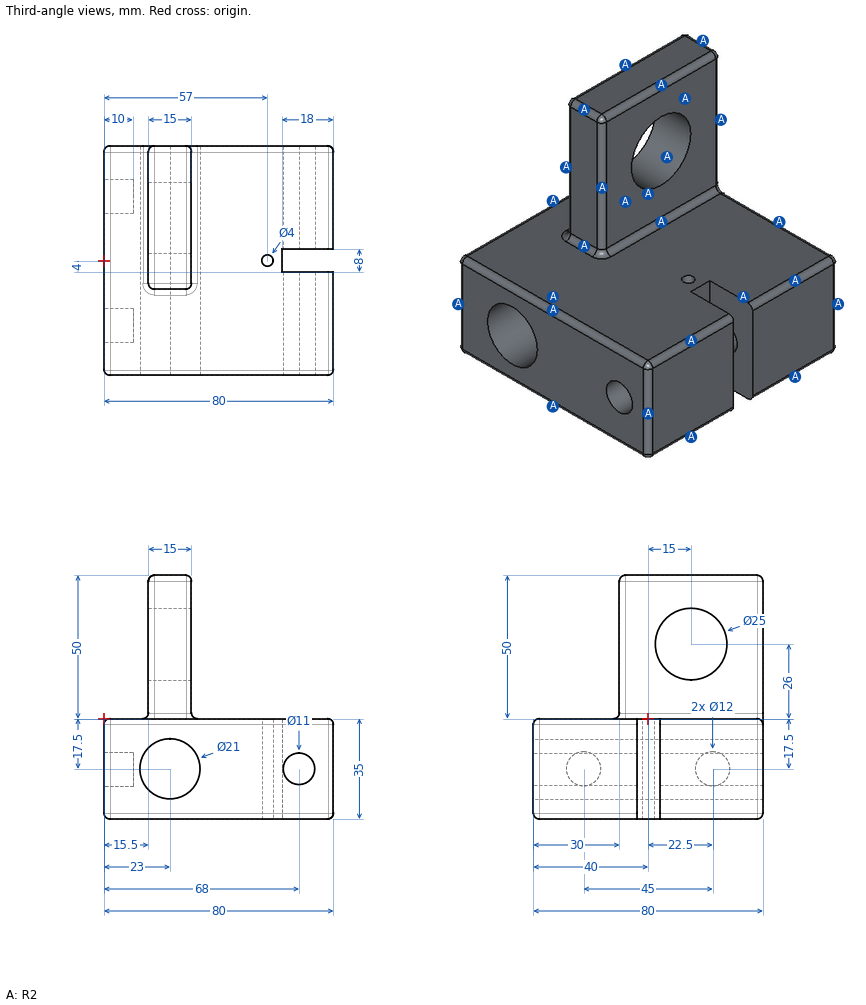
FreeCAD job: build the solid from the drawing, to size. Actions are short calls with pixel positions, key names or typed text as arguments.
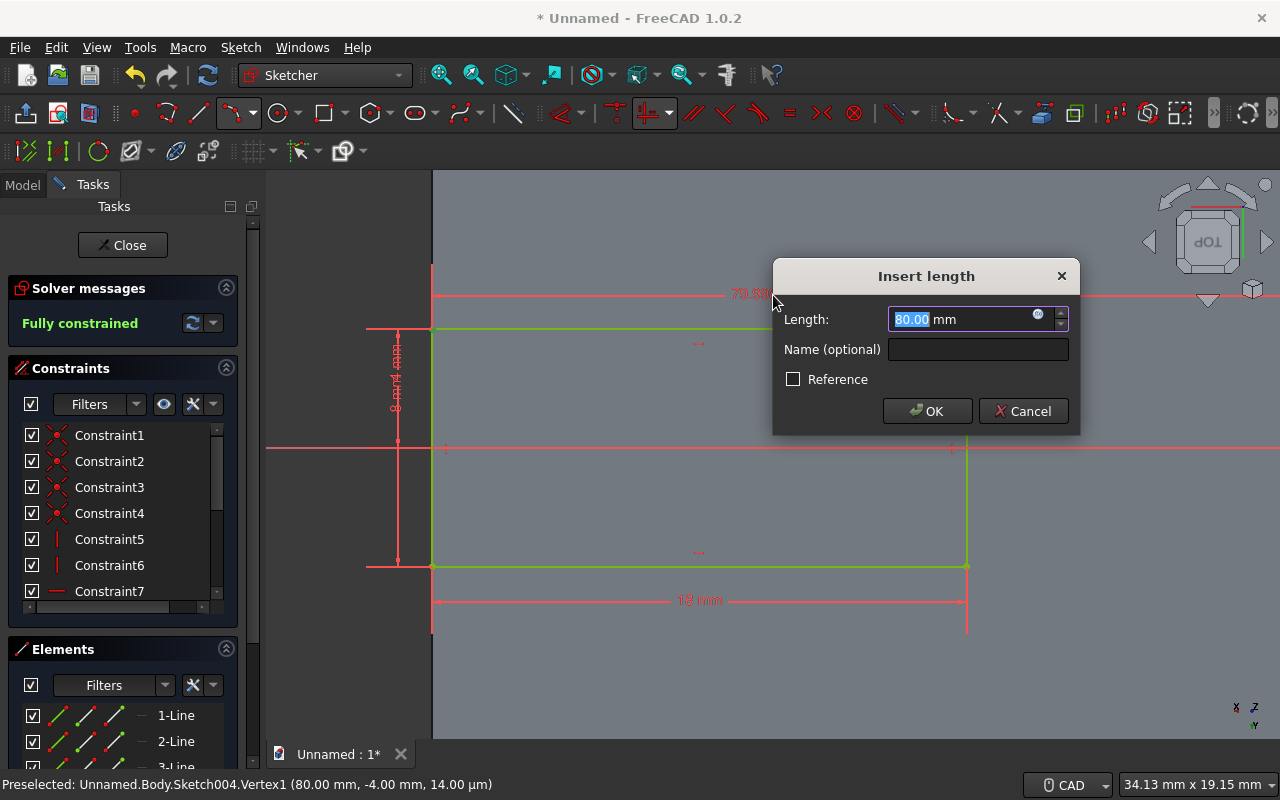
text(80)
key(Return)
key(Escape)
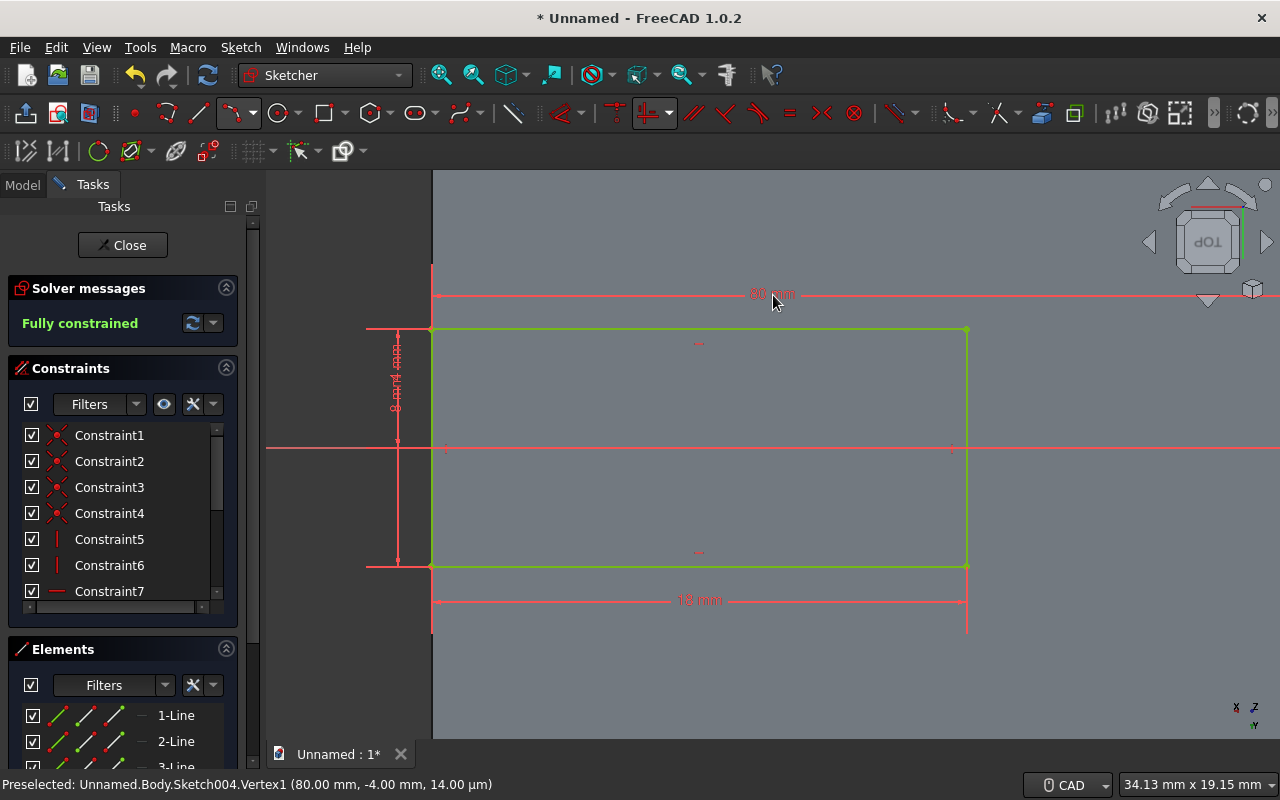
click(123, 245)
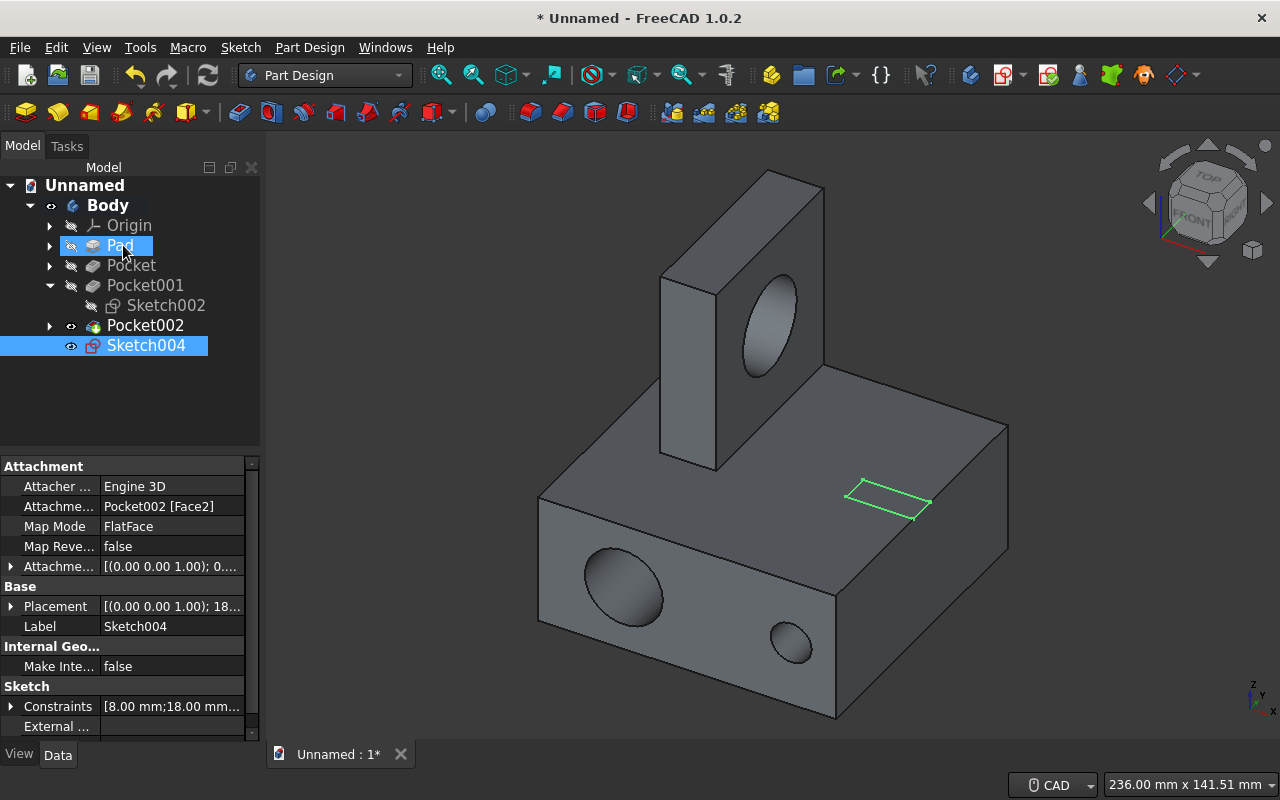
click(240, 112)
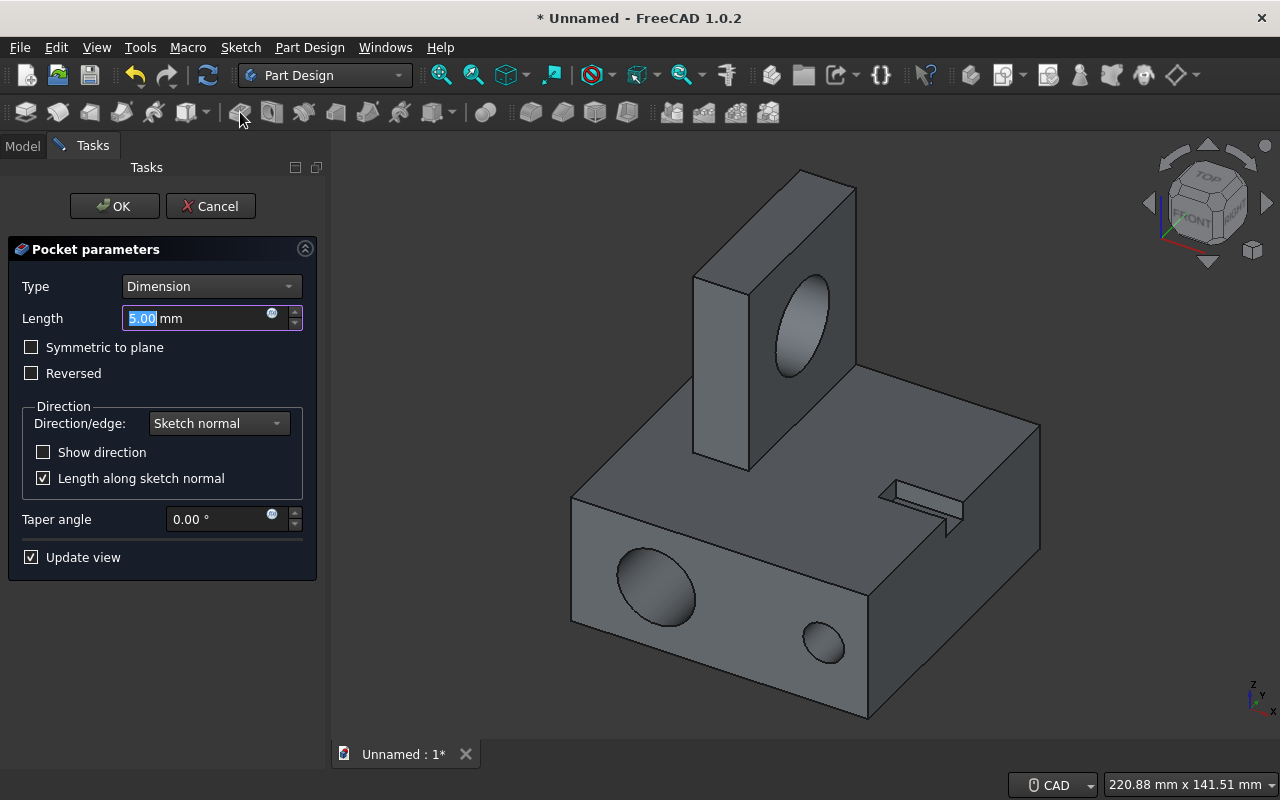
click(212, 286)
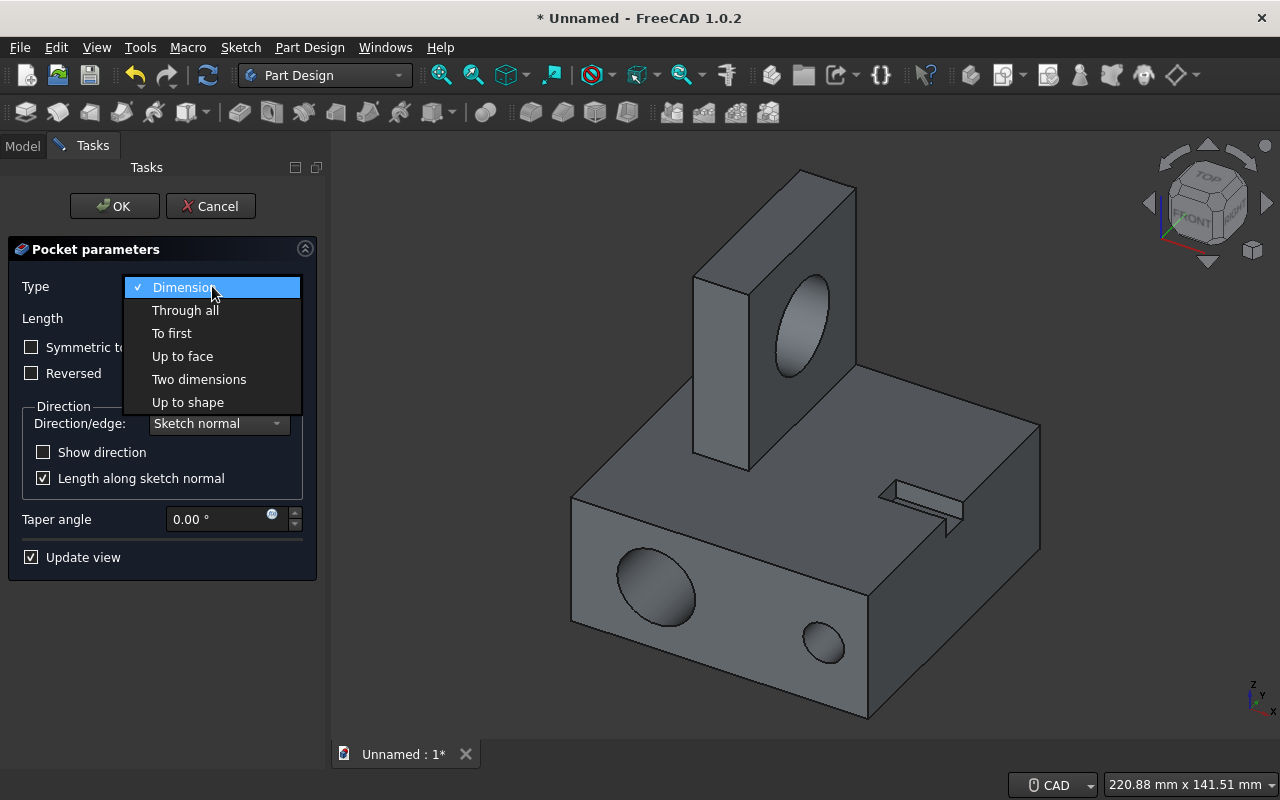
click(212, 310)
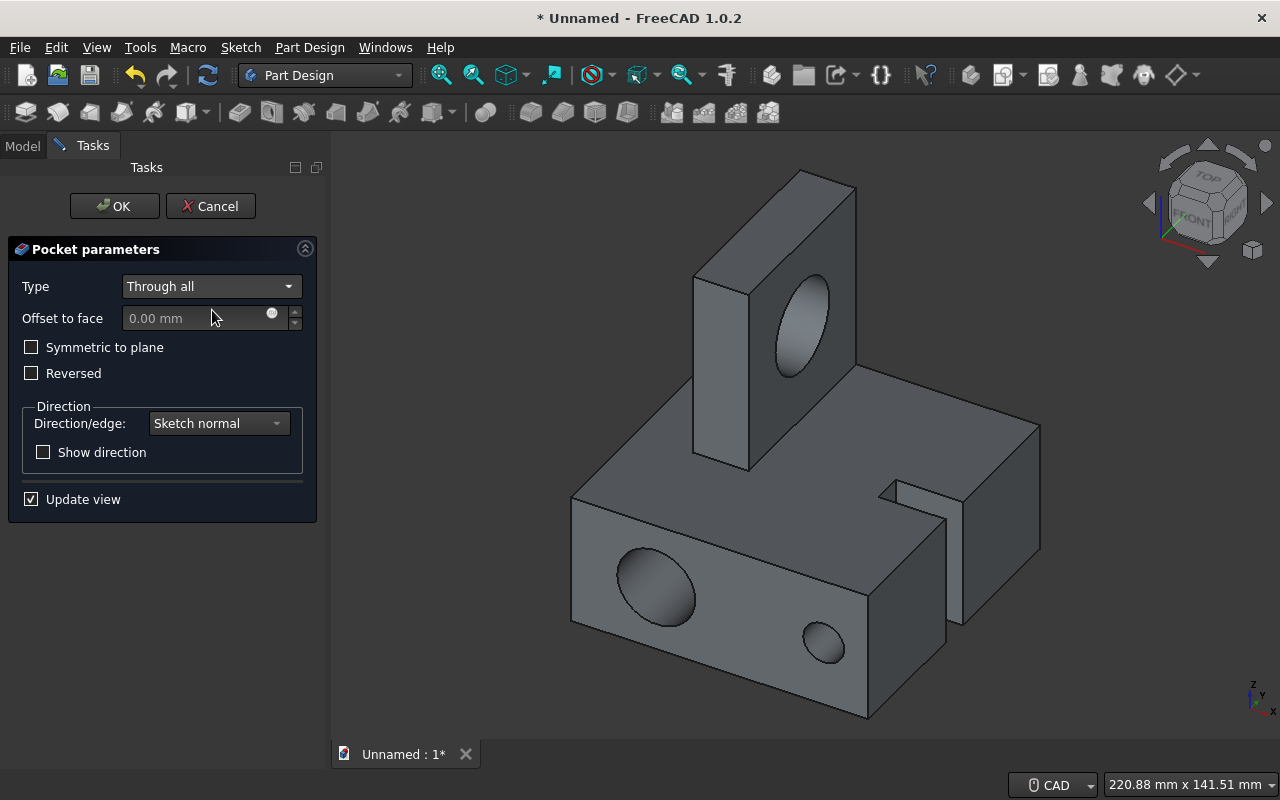
click(115, 206)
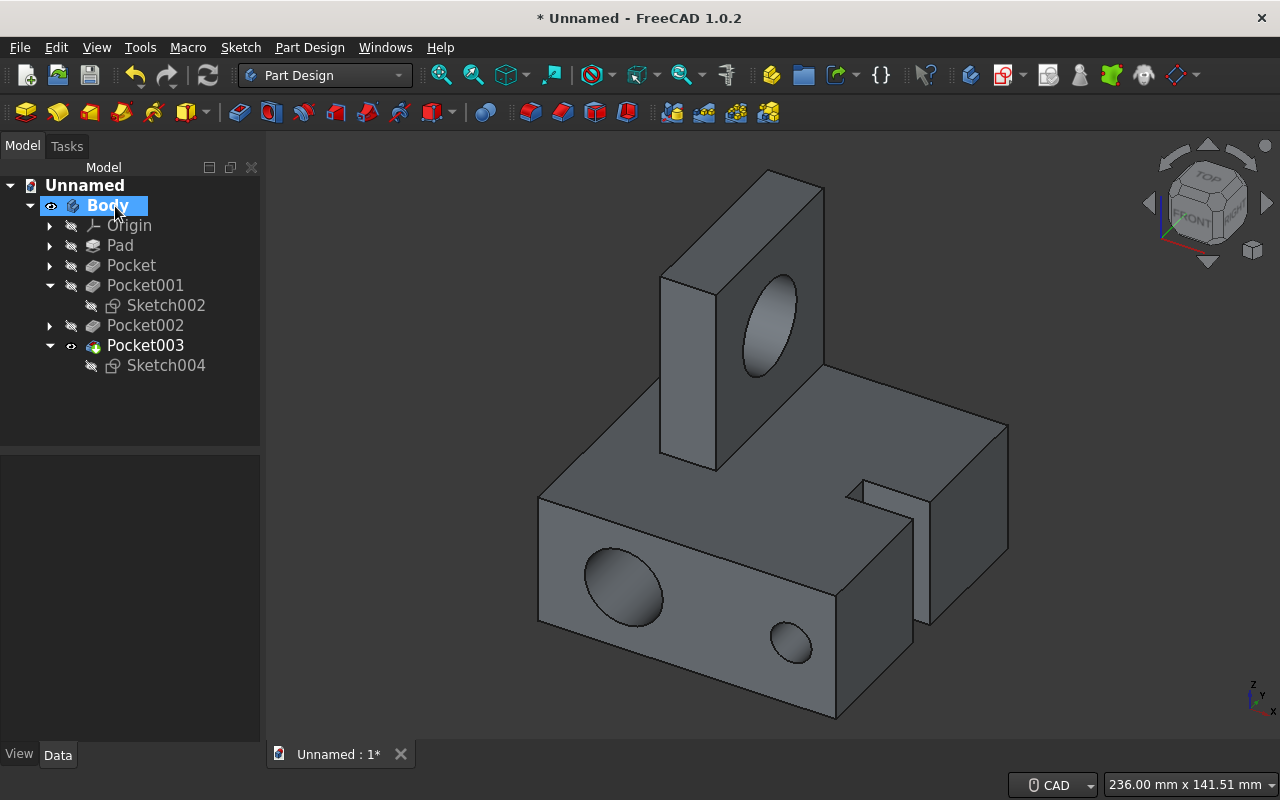
click(773, 201)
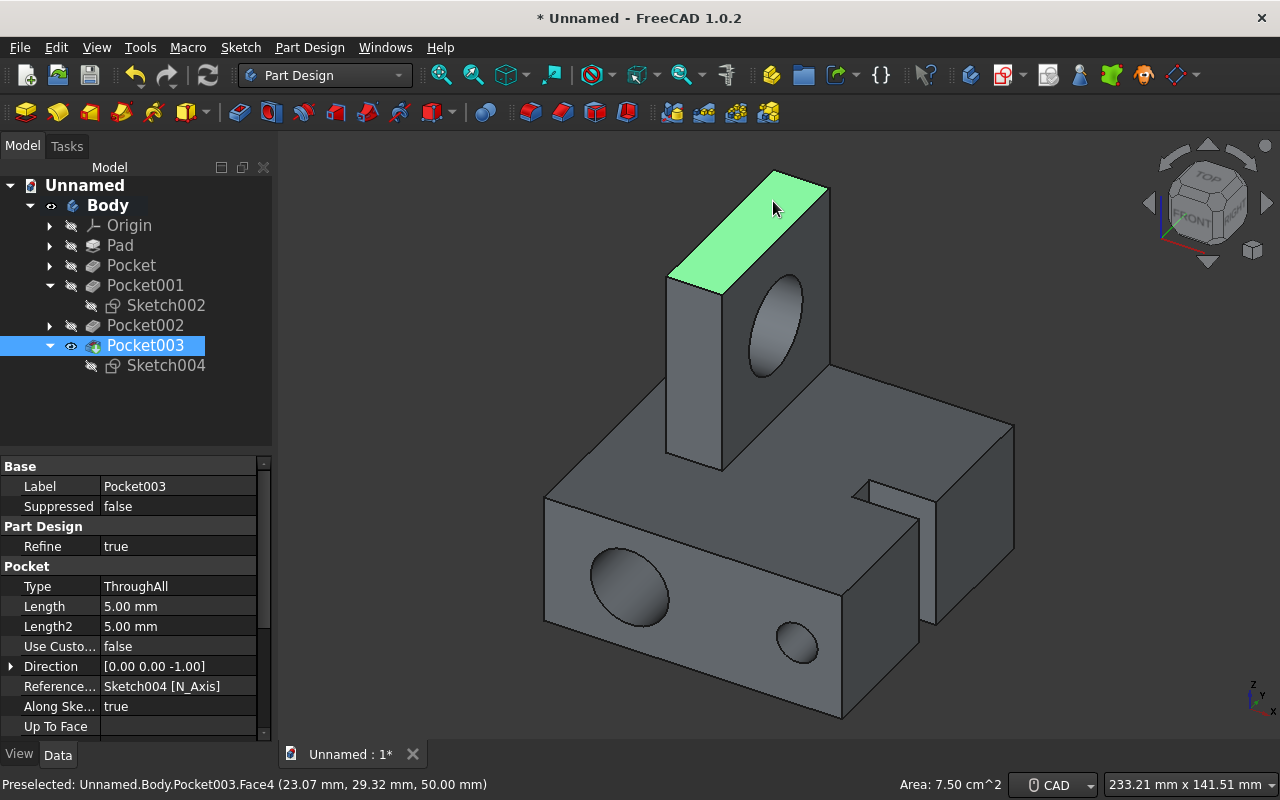
click(694, 323, ctrl)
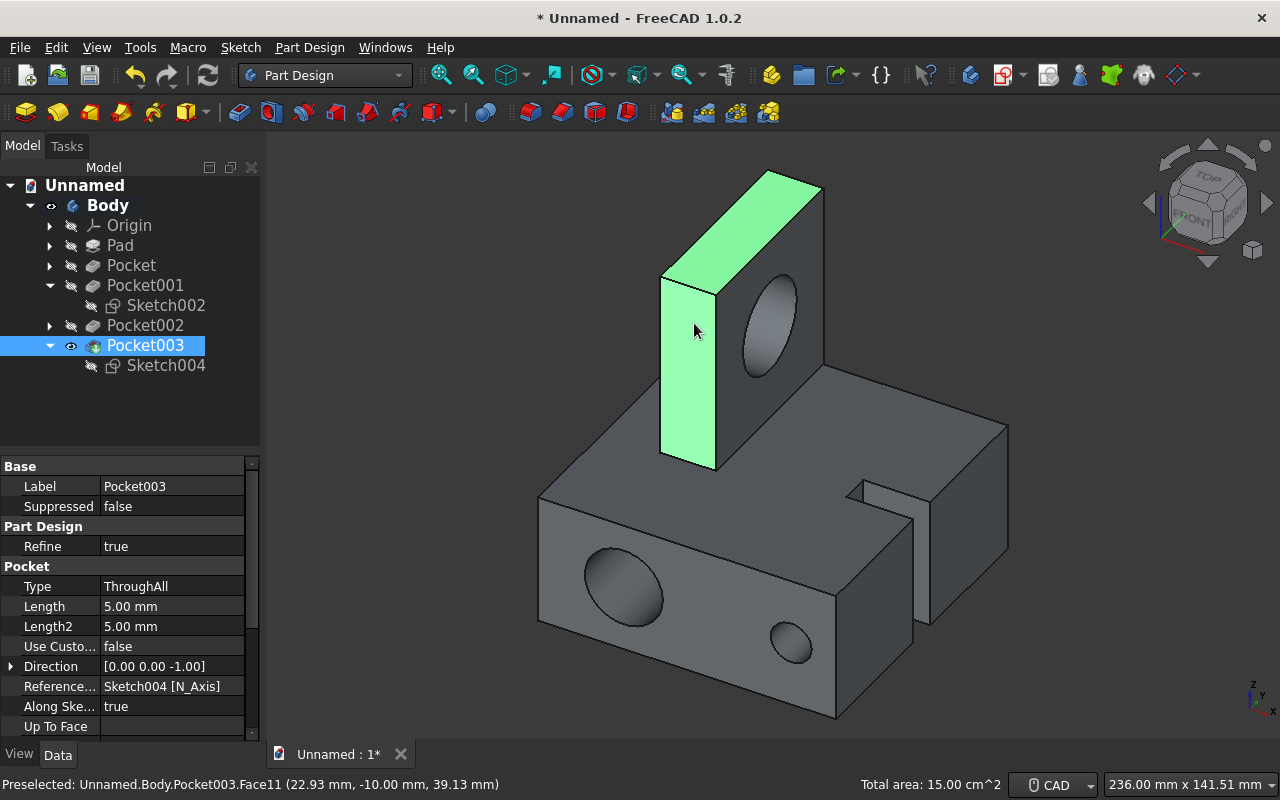
click(687, 546, ctrl)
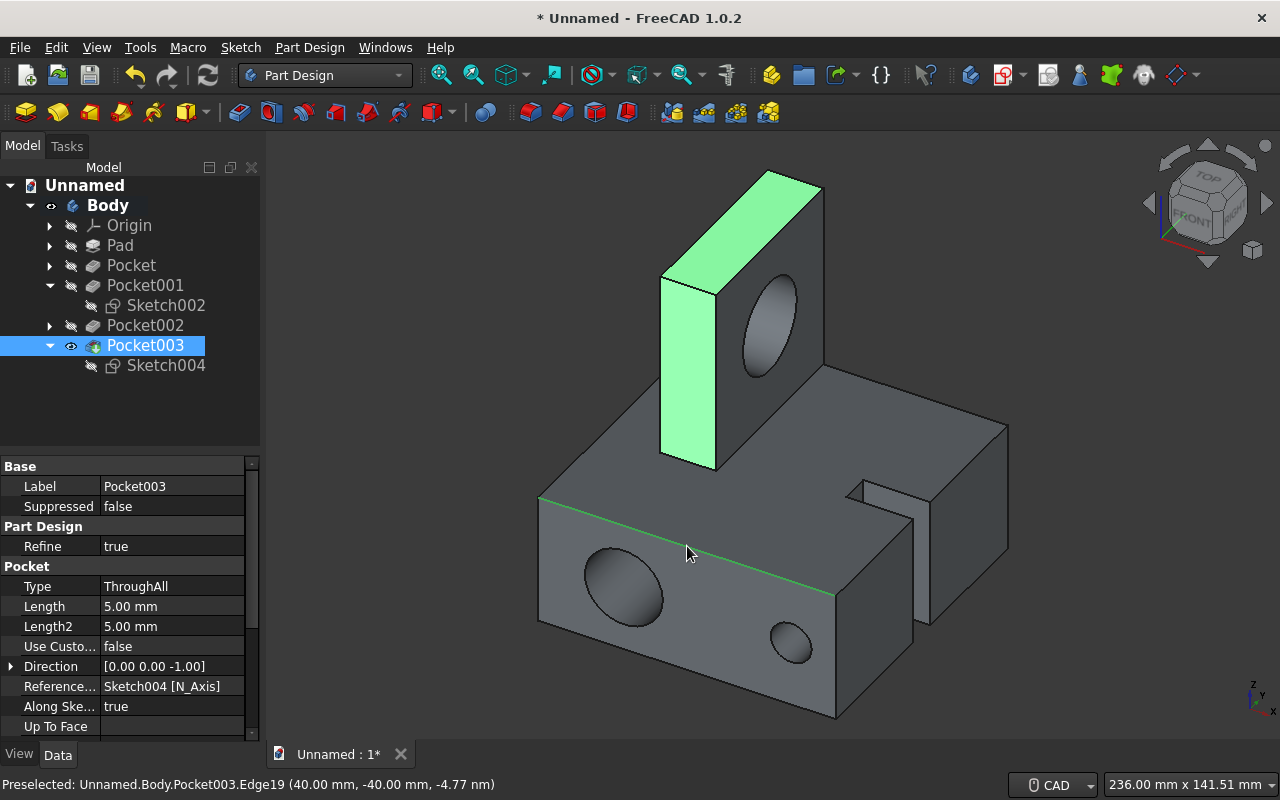
click(836, 657, ctrl)